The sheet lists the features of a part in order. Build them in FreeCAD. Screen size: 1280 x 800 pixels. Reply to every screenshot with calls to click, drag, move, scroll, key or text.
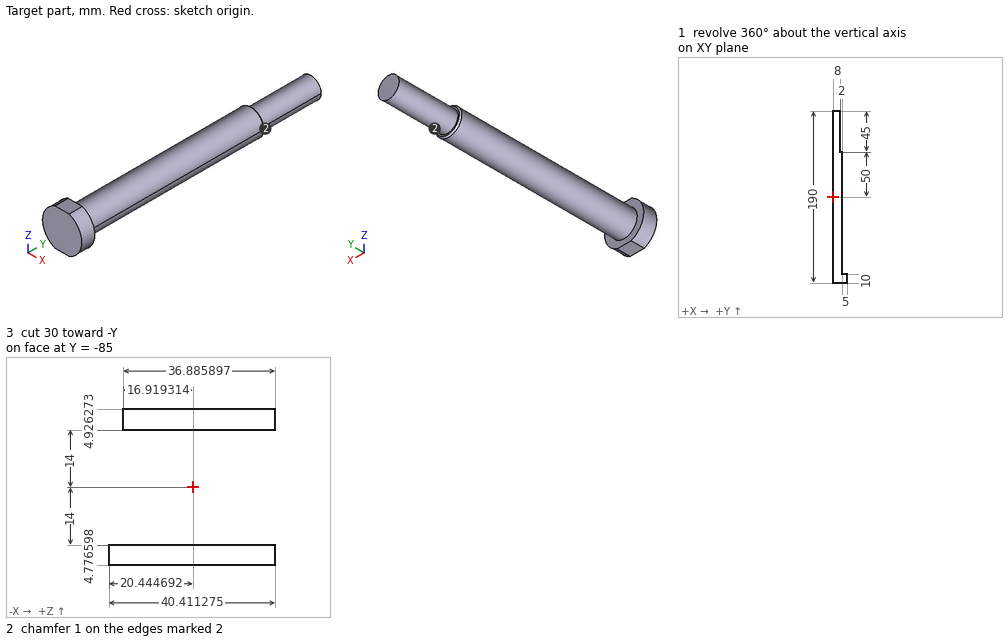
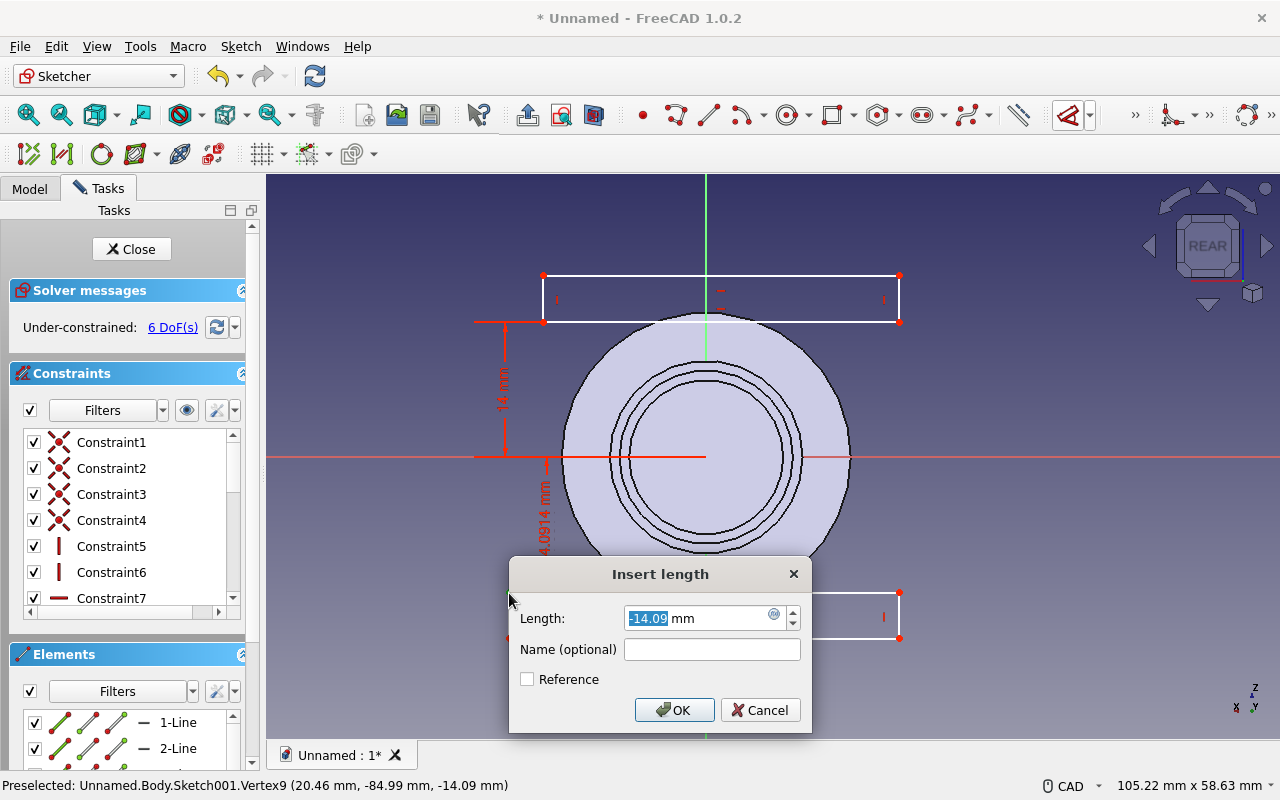
text(-14)
key(Return)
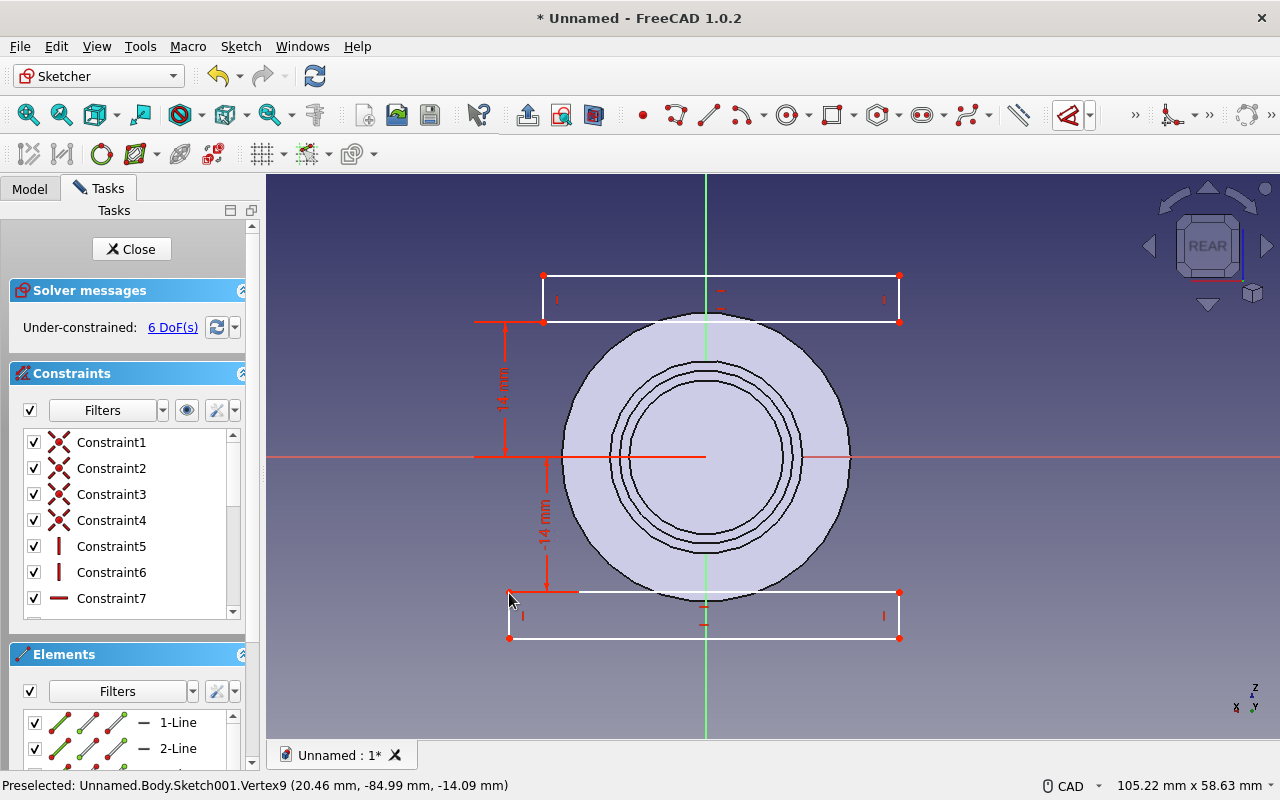
click(543, 290)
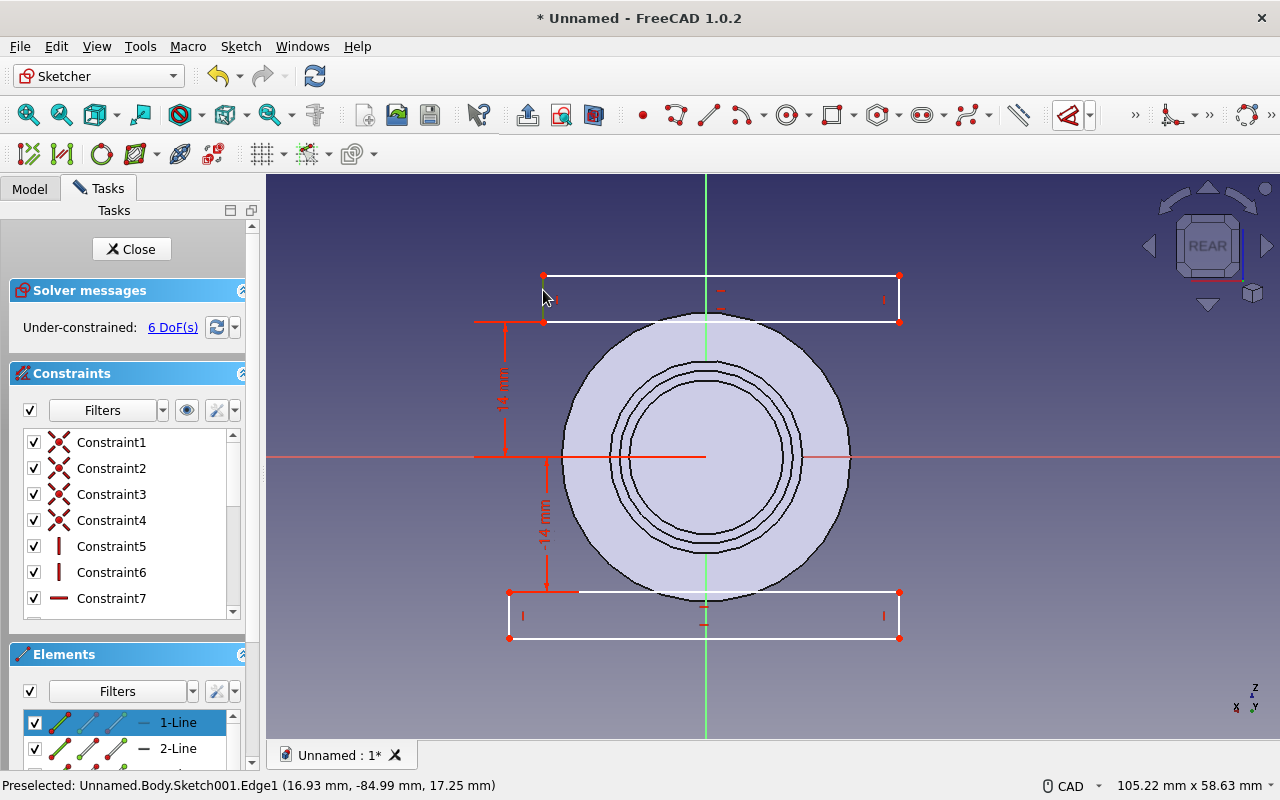
click(1090, 116)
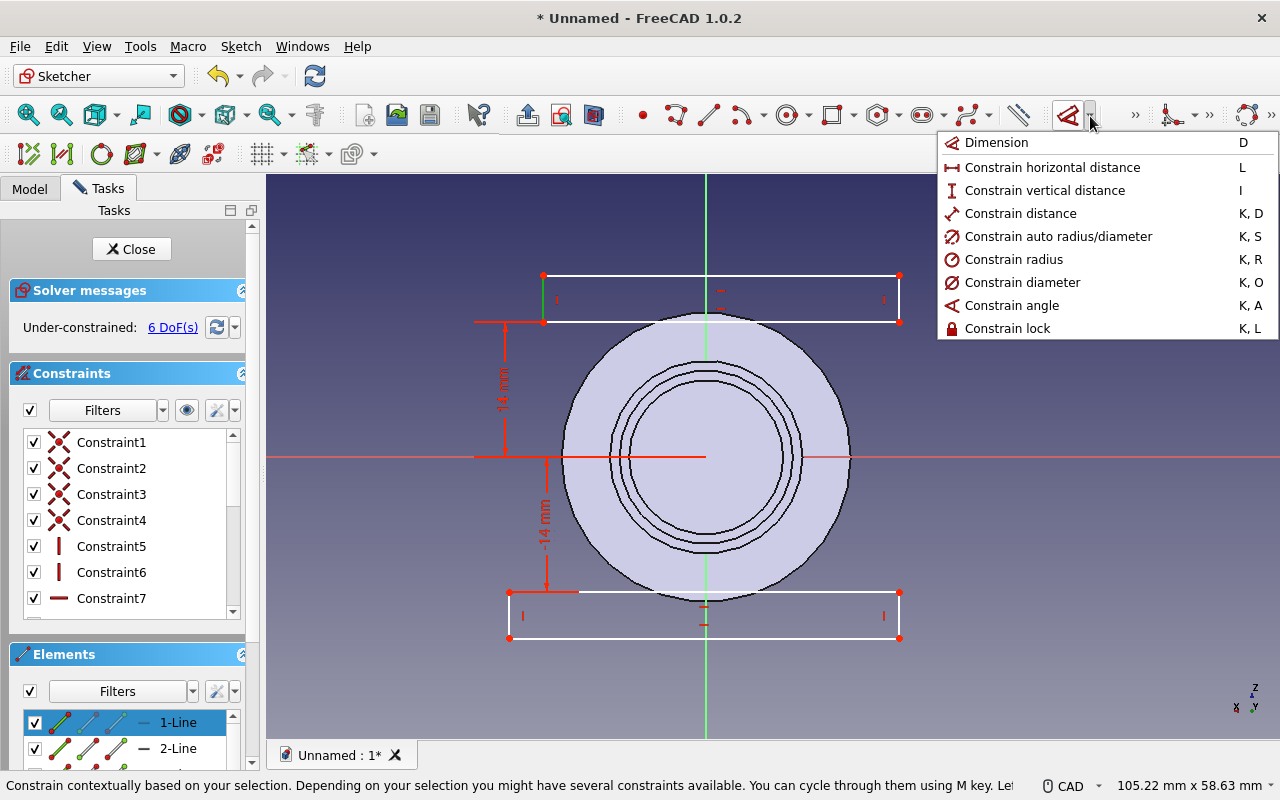
click(1108, 190)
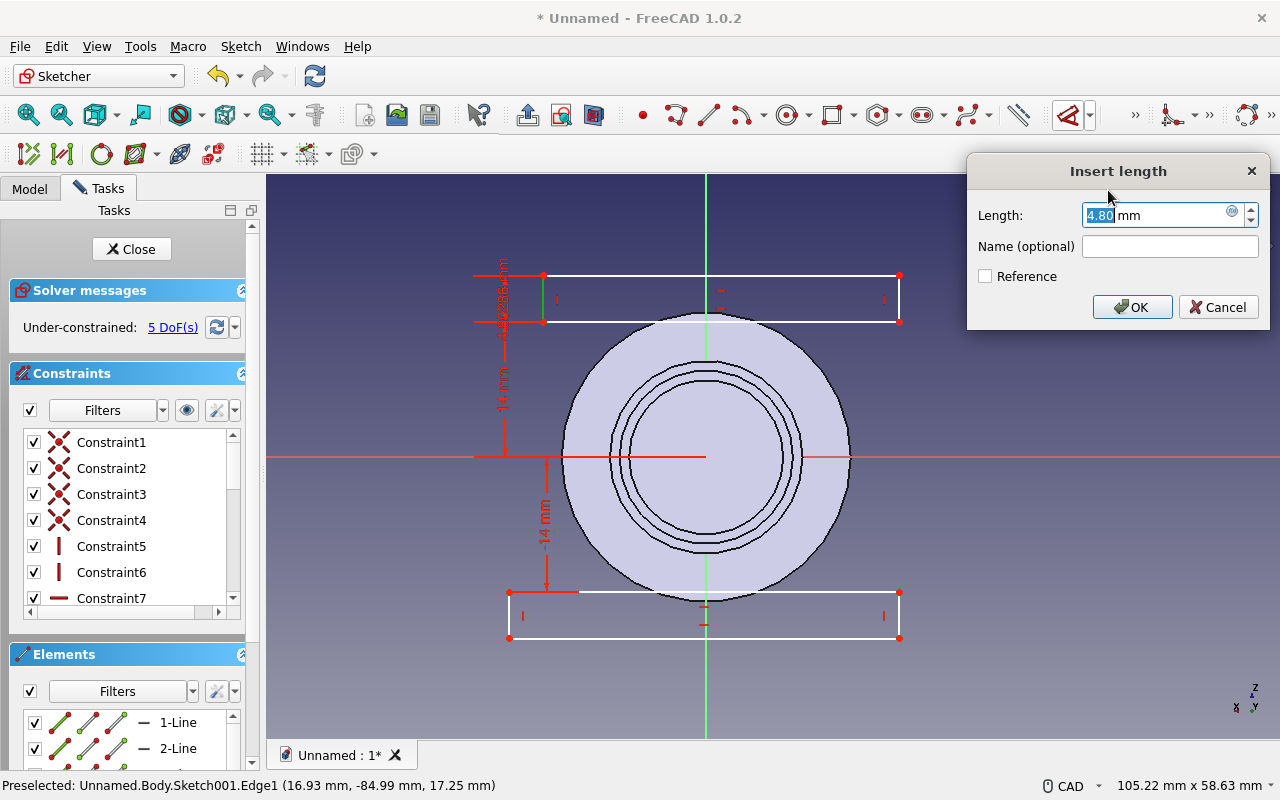
text(4.926273)
key(Return)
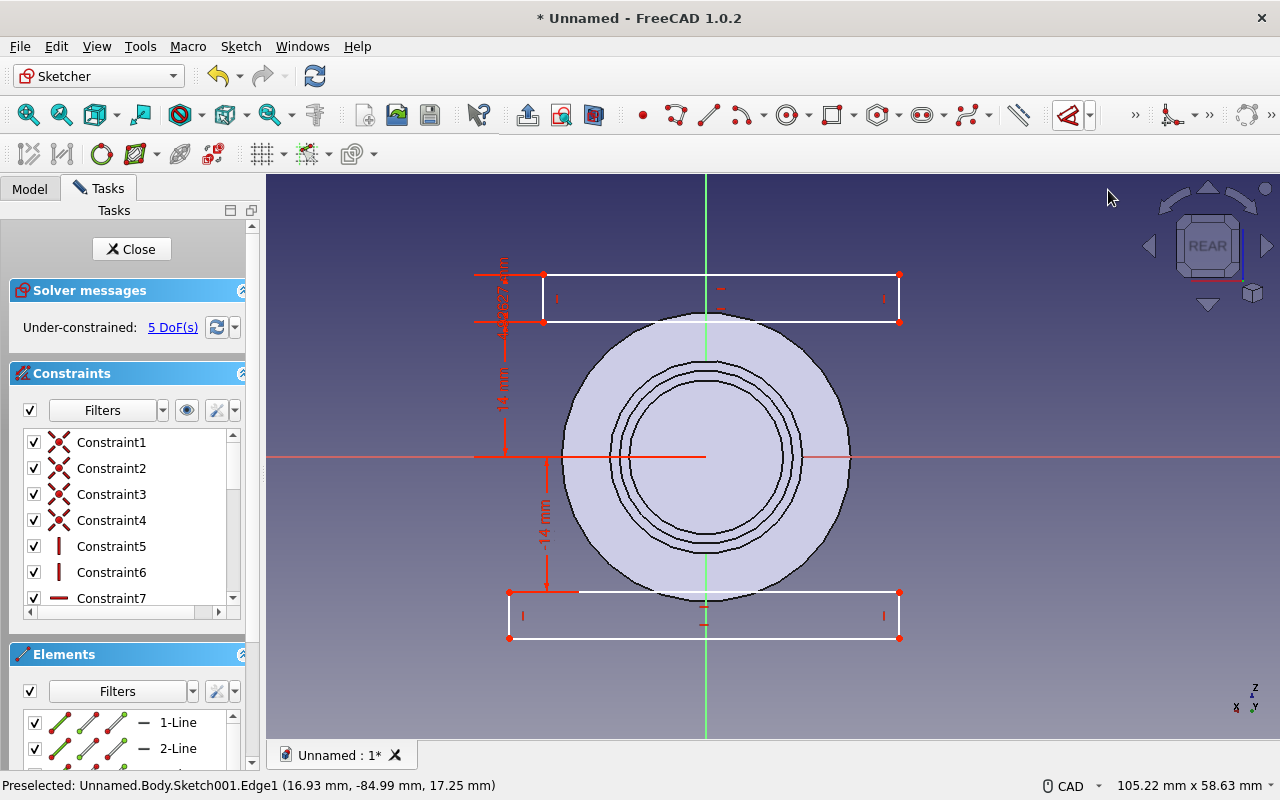
click(509, 606)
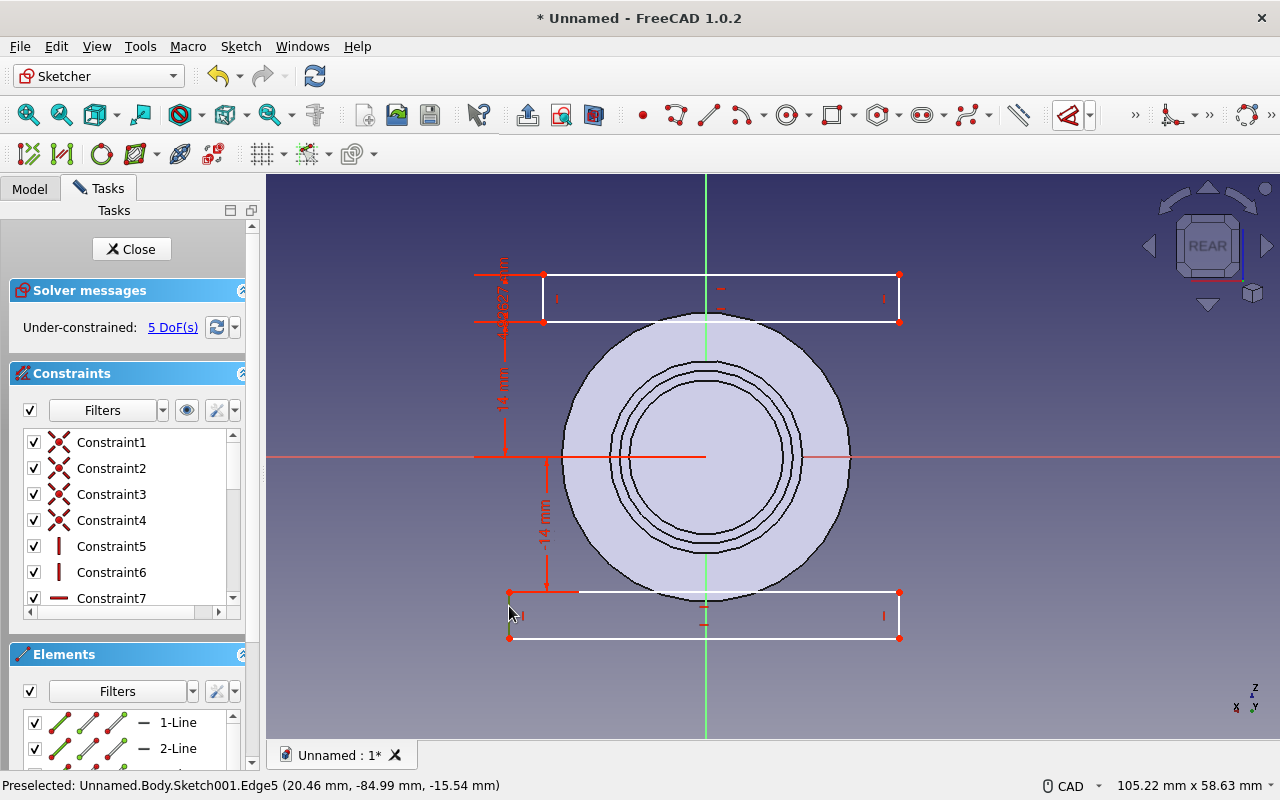
key(i)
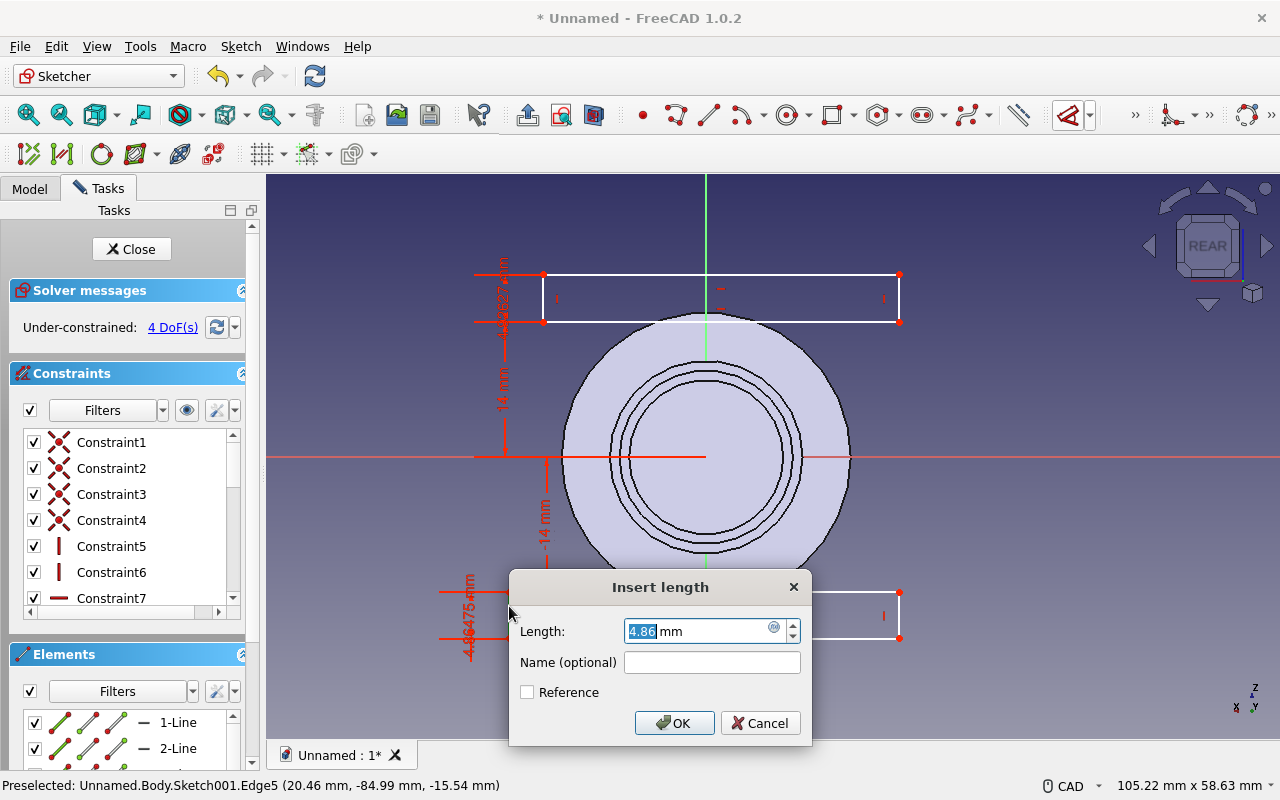
text(4.776598)
key(Return)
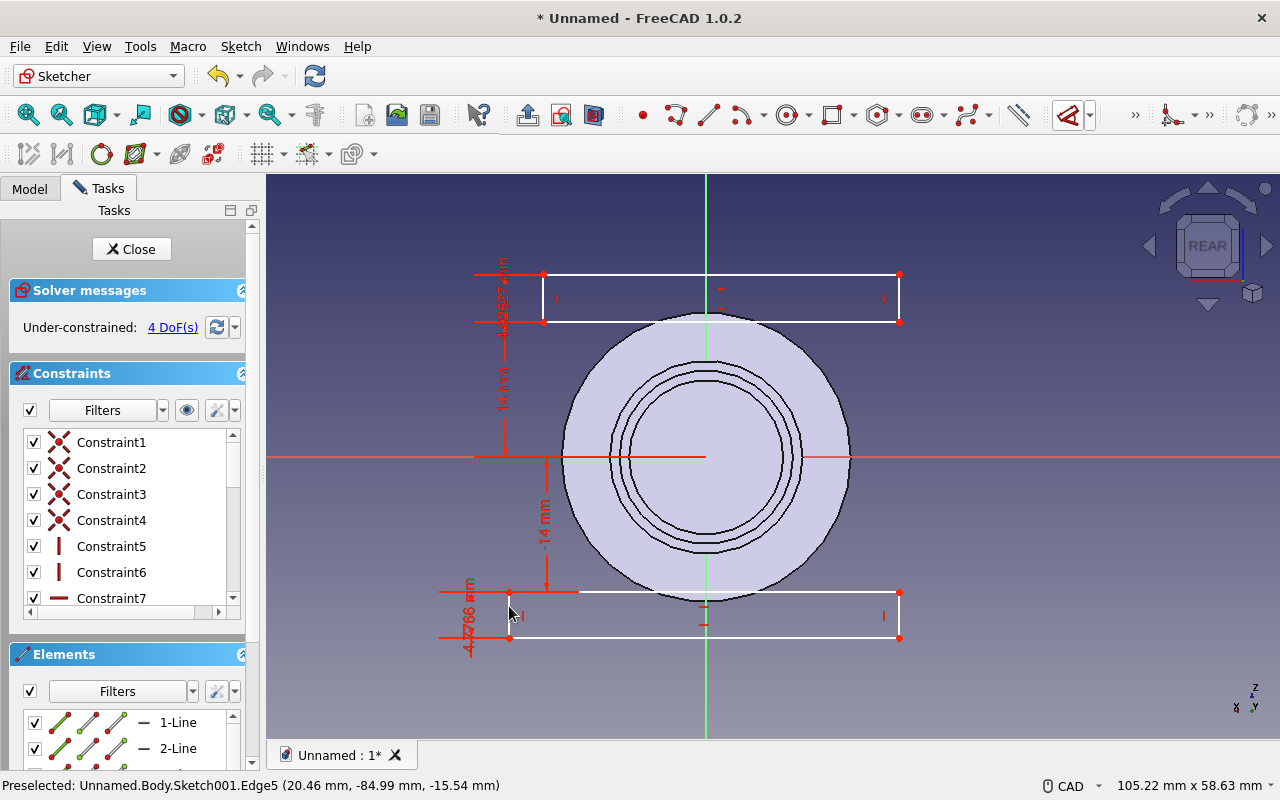
click(650, 322)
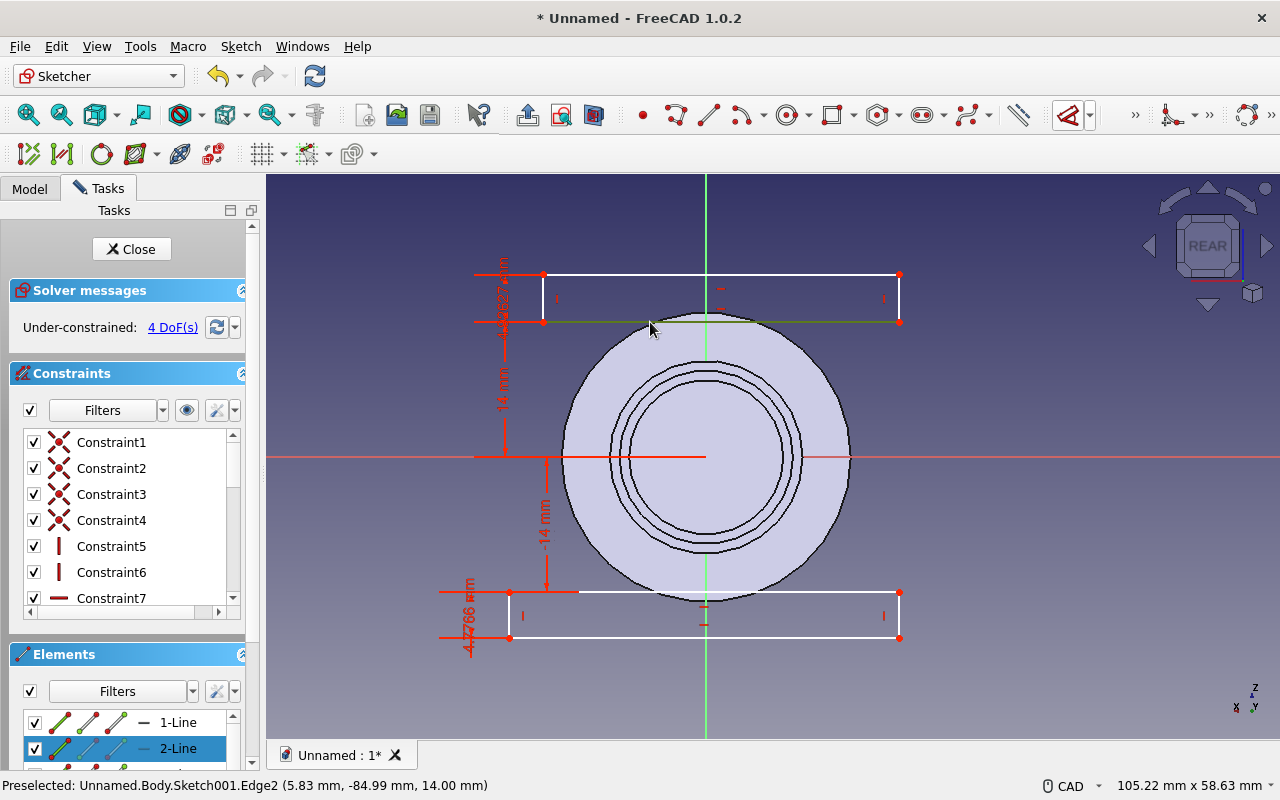
key(l)